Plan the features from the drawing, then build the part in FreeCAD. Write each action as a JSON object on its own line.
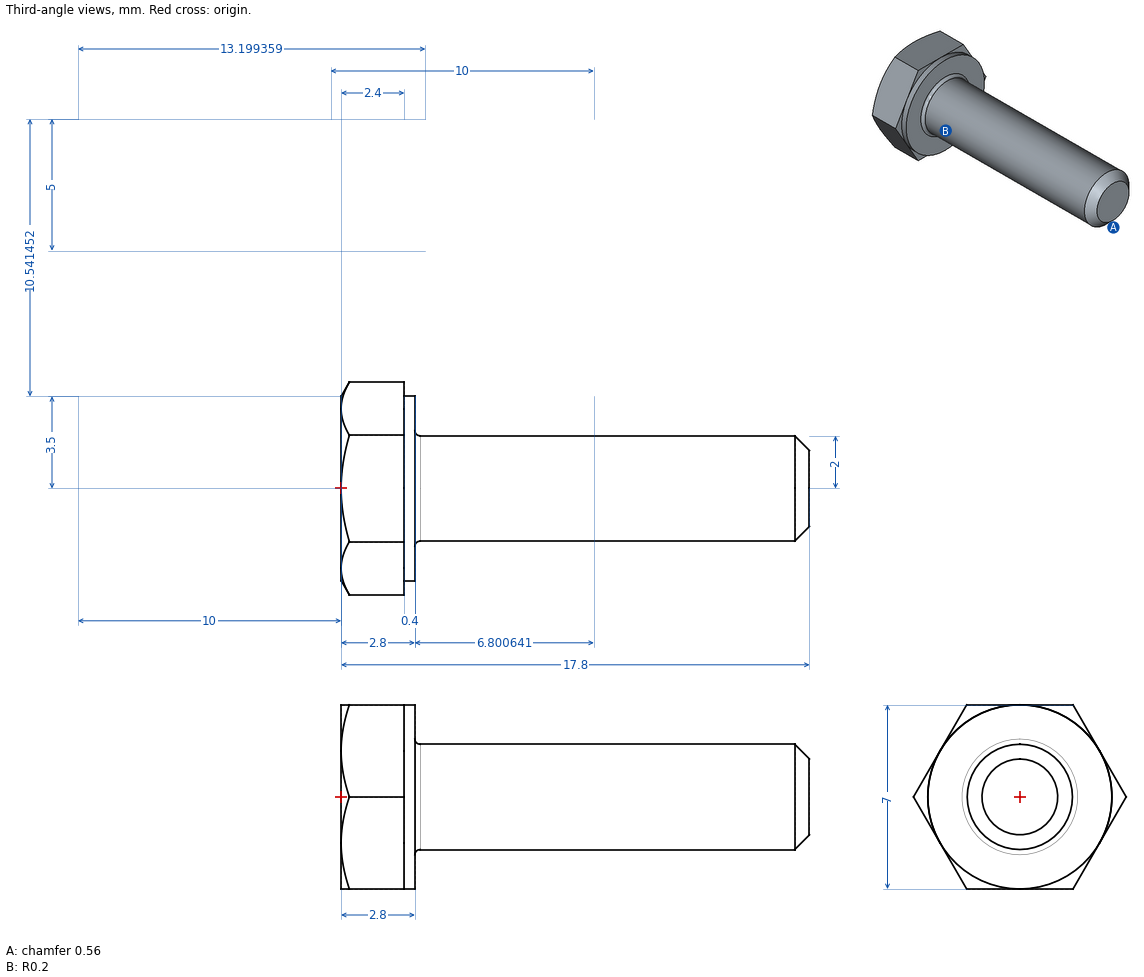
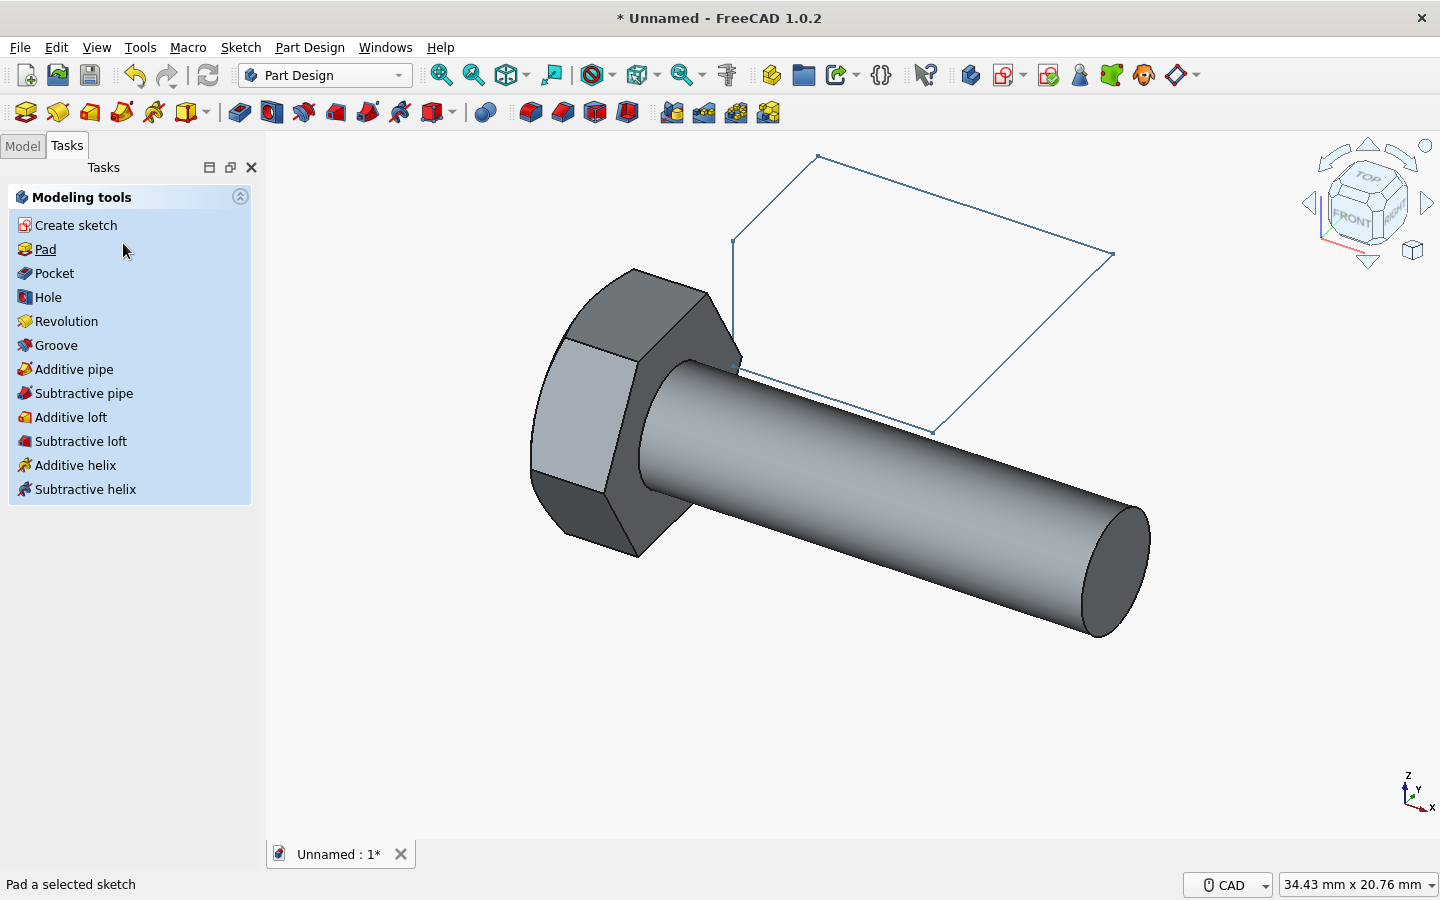
{"action": "left_click", "coordinate": [304, 112]}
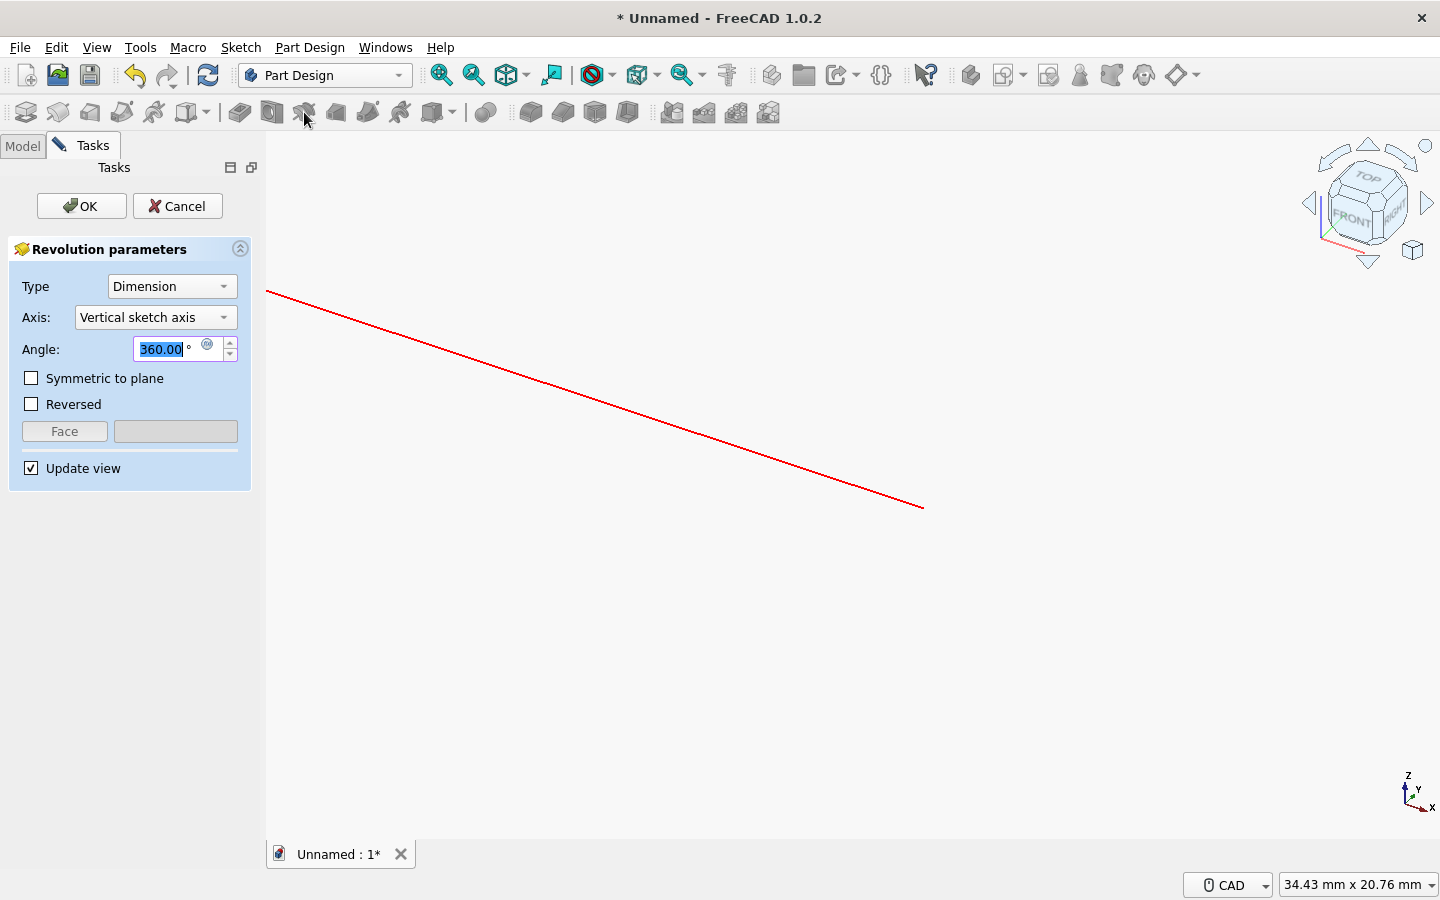
{"action": "left_click", "coordinate": [156, 318]}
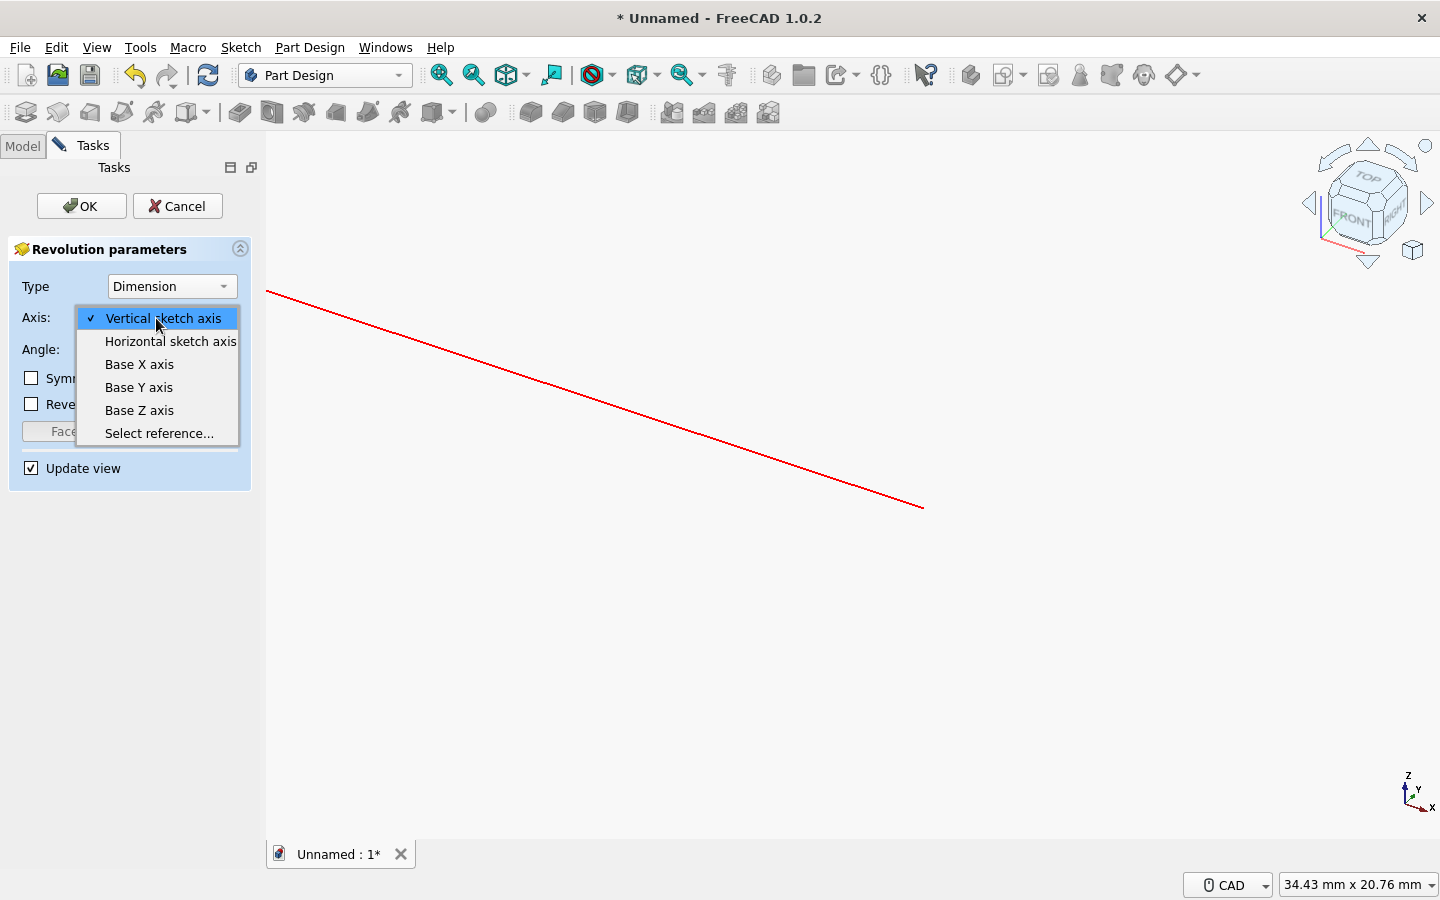
{"action": "left_click", "coordinate": [156, 342]}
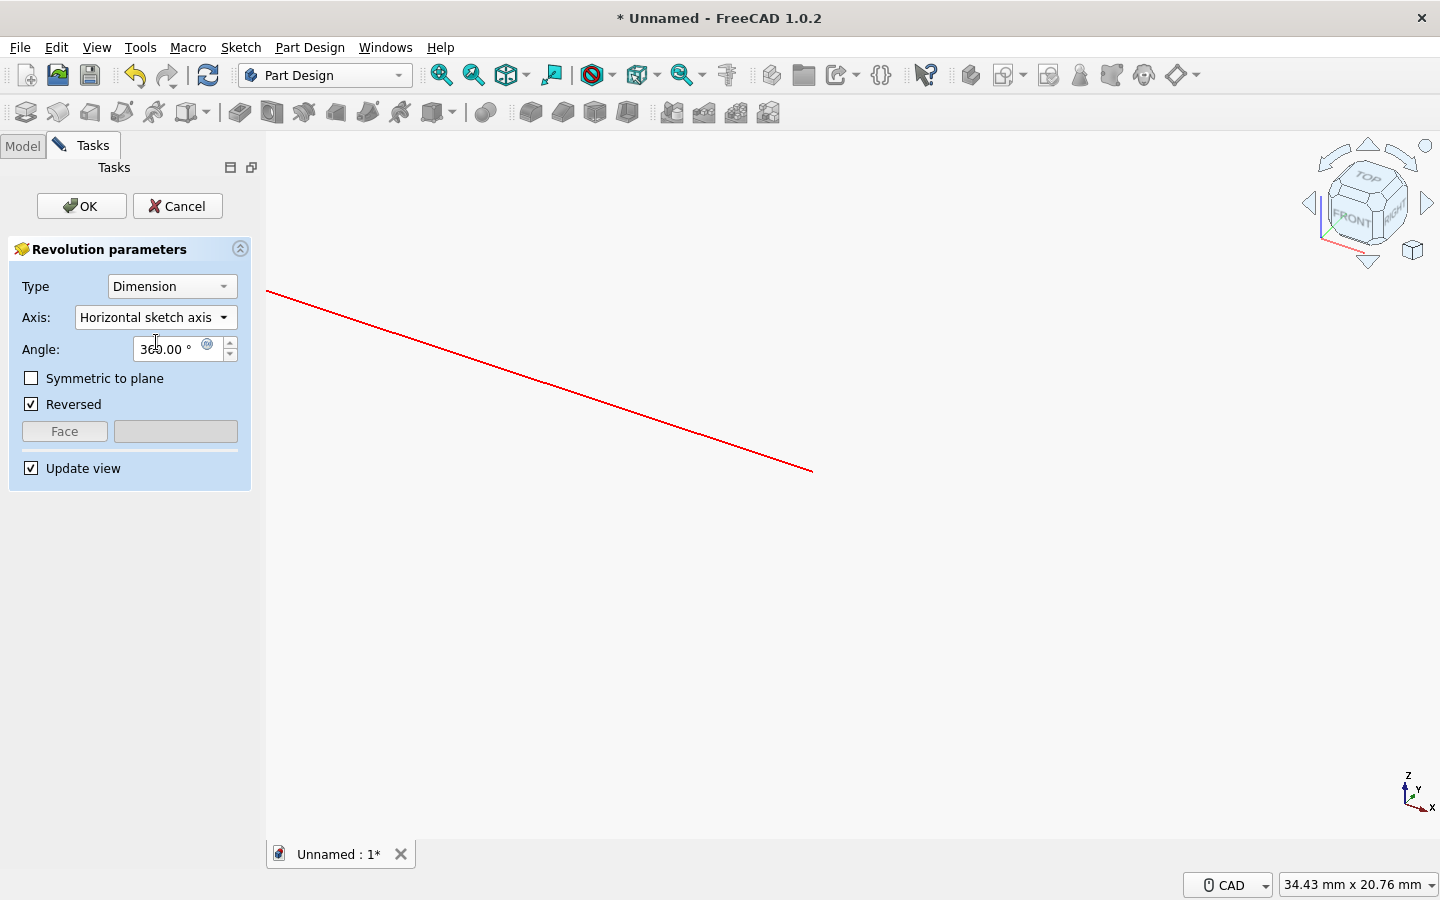
{"action": "left_click", "coordinate": [82, 206]}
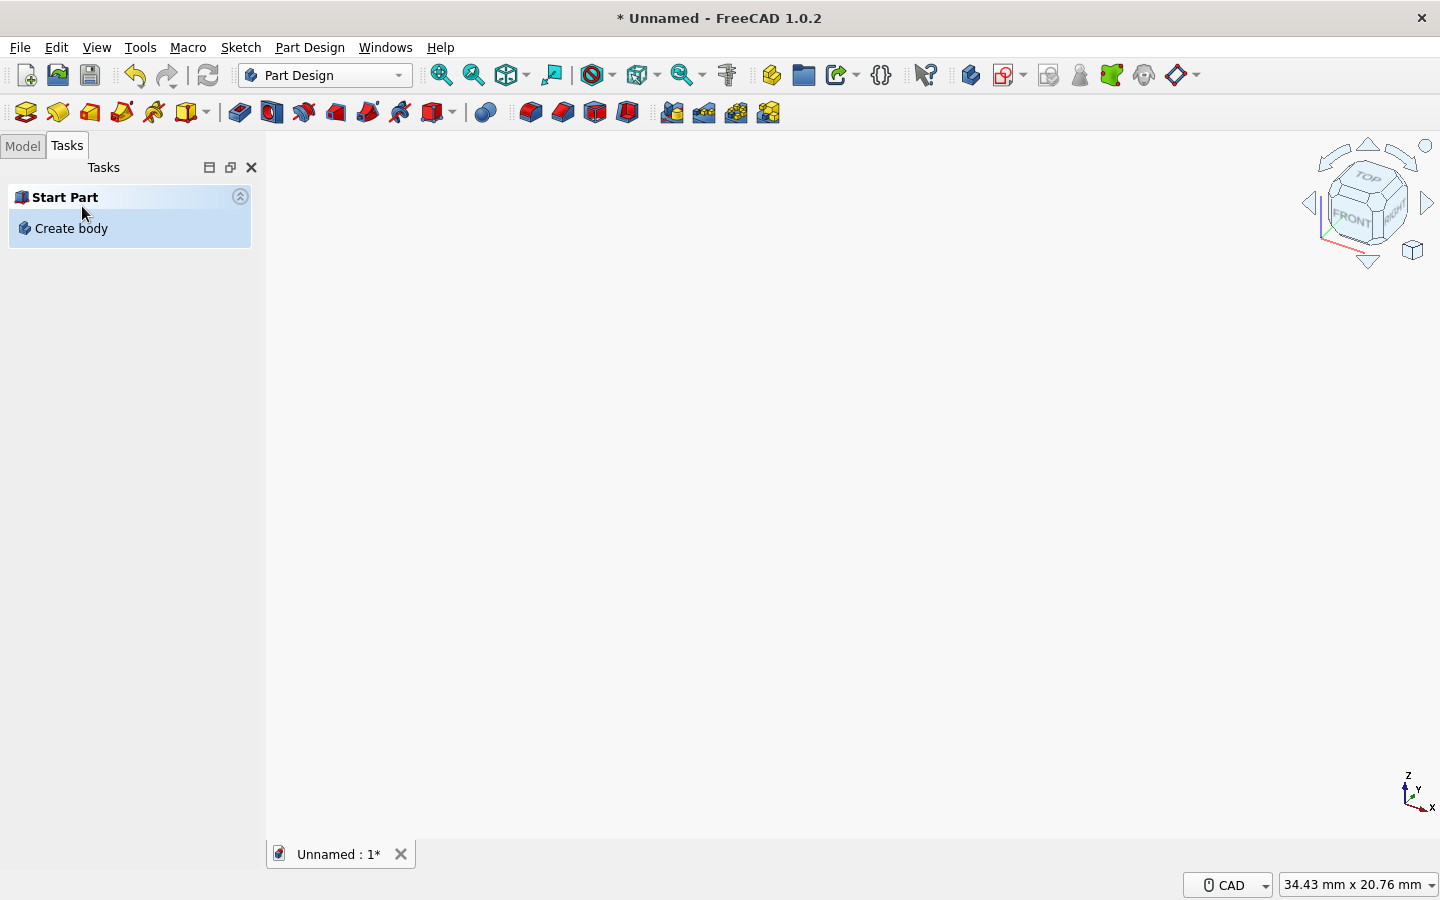
{"action": "key", "text": "v f"}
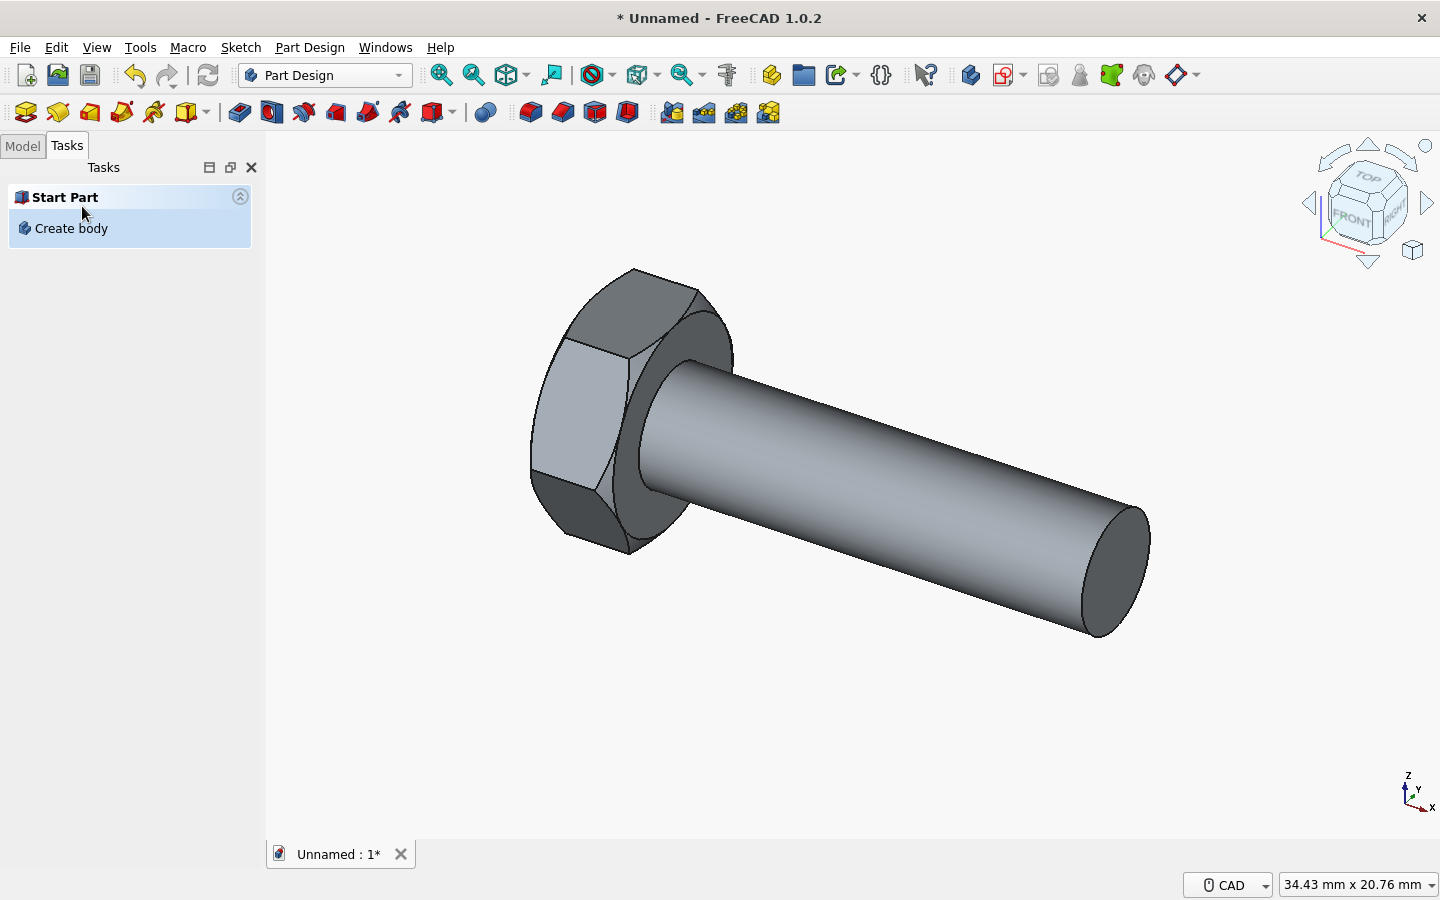
{"action": "left_click", "coordinate": [1004, 76]}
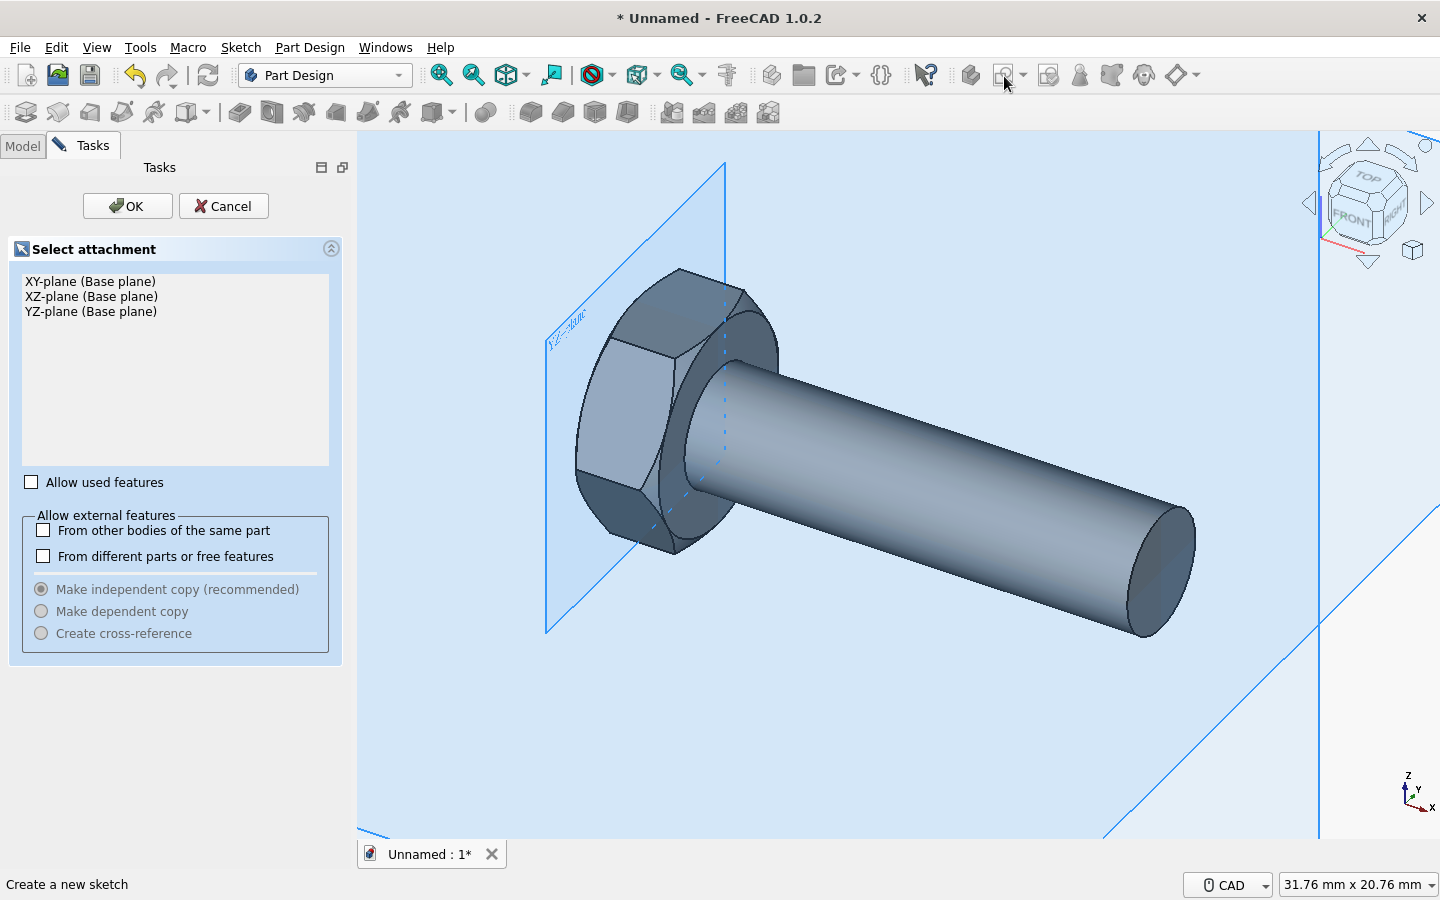
{"action": "left_click", "coordinate": [82, 282]}